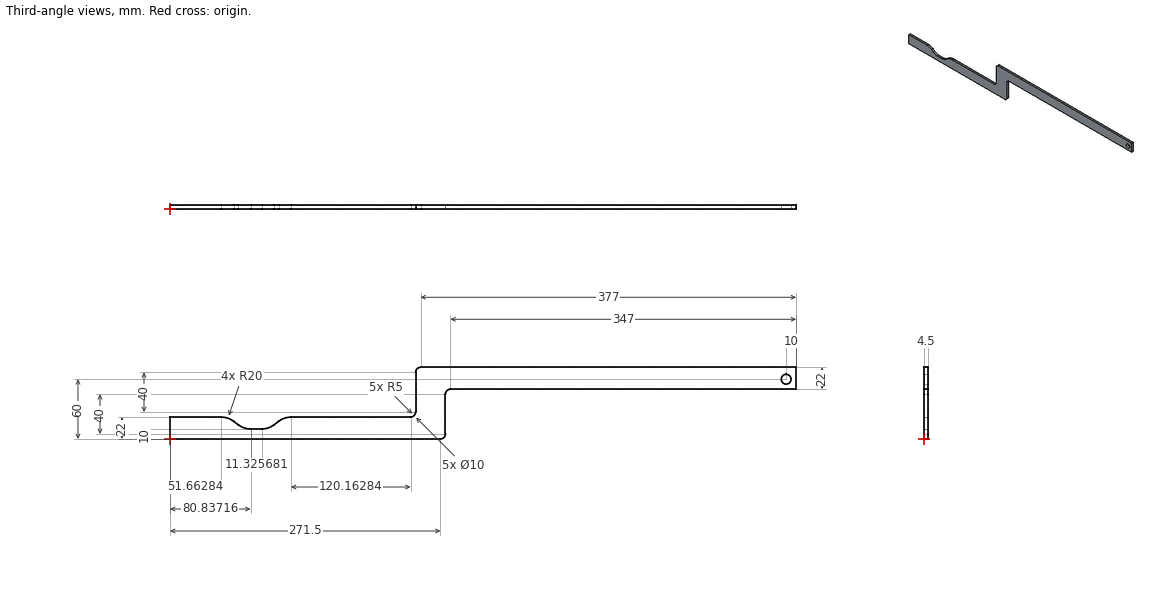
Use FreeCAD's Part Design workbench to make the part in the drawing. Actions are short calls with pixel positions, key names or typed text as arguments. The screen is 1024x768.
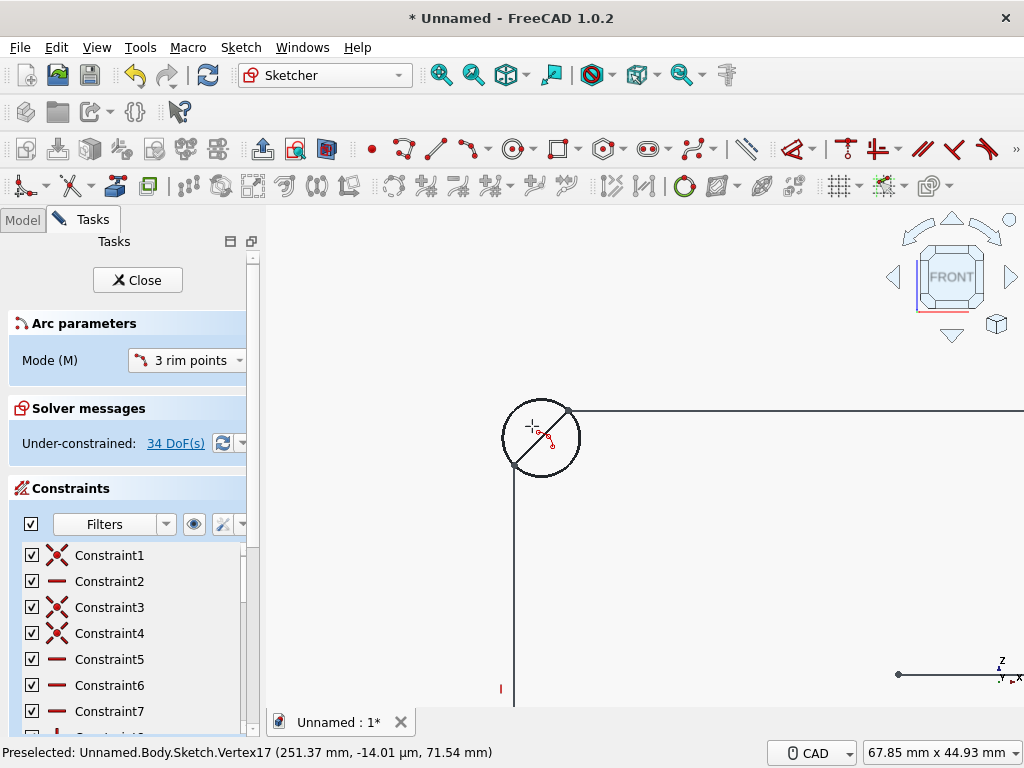
click(530, 422)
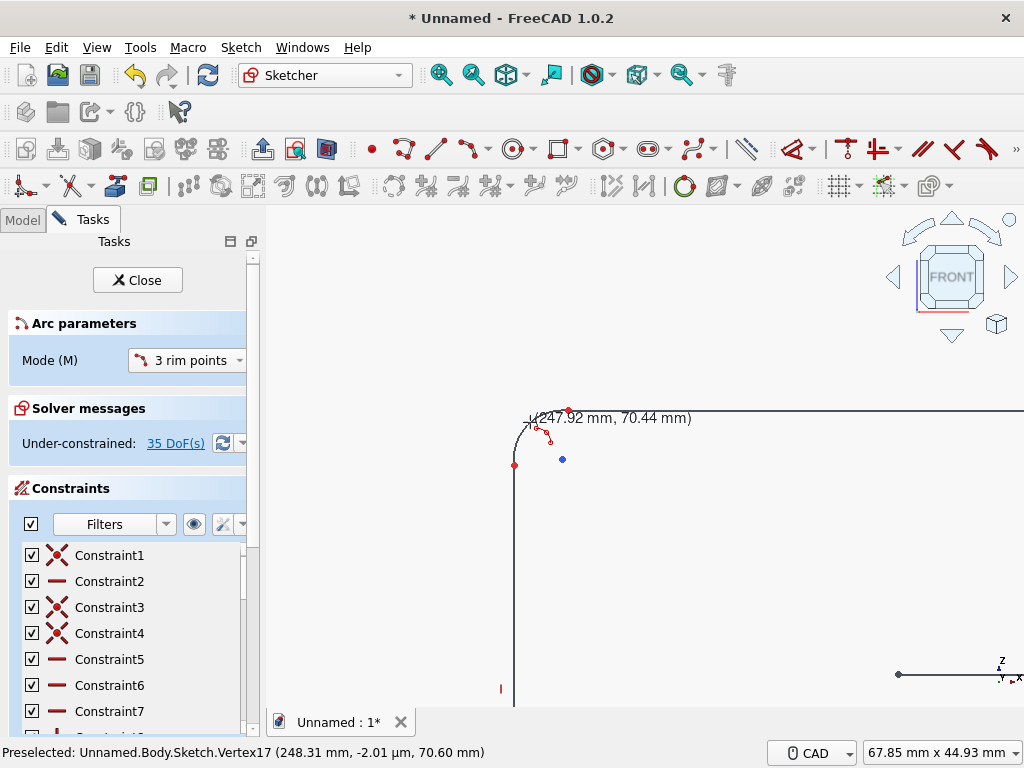
scroll(532, 433, down, 14)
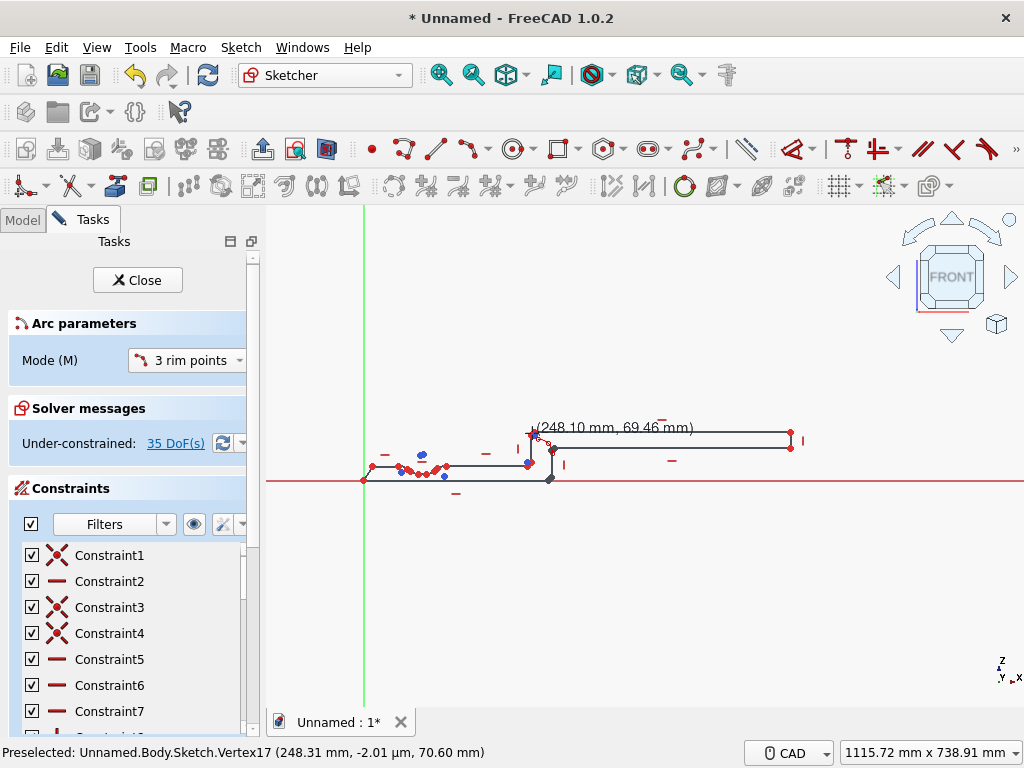
scroll(555, 447, up, 6)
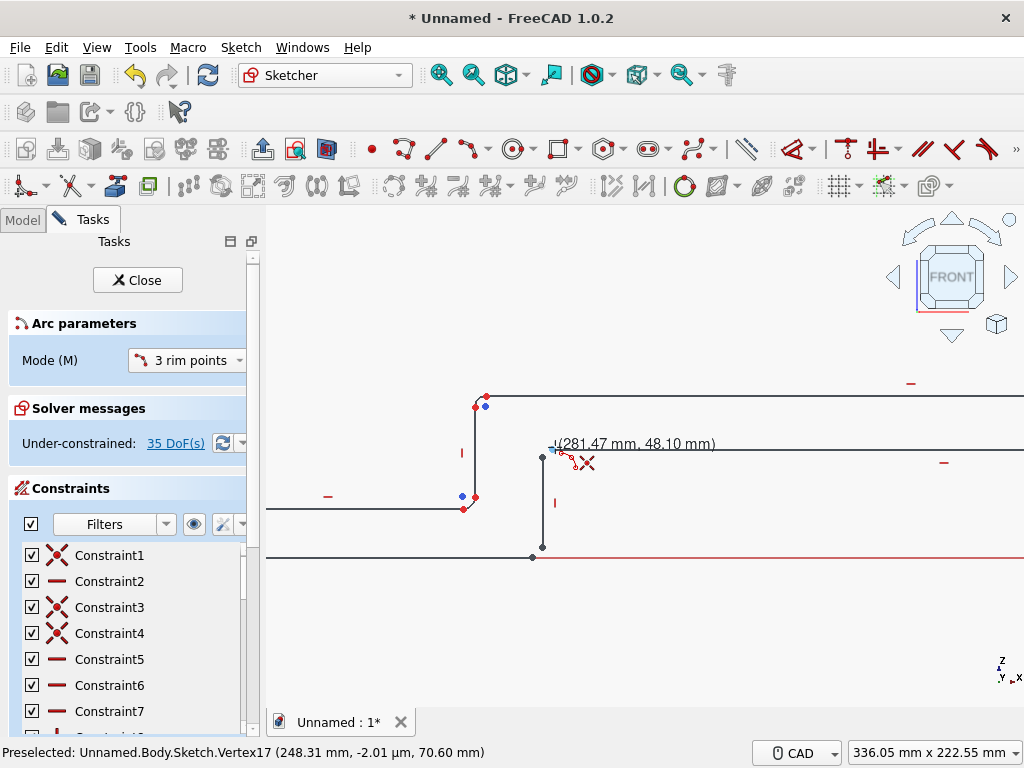
click(553, 450)
click(543, 457)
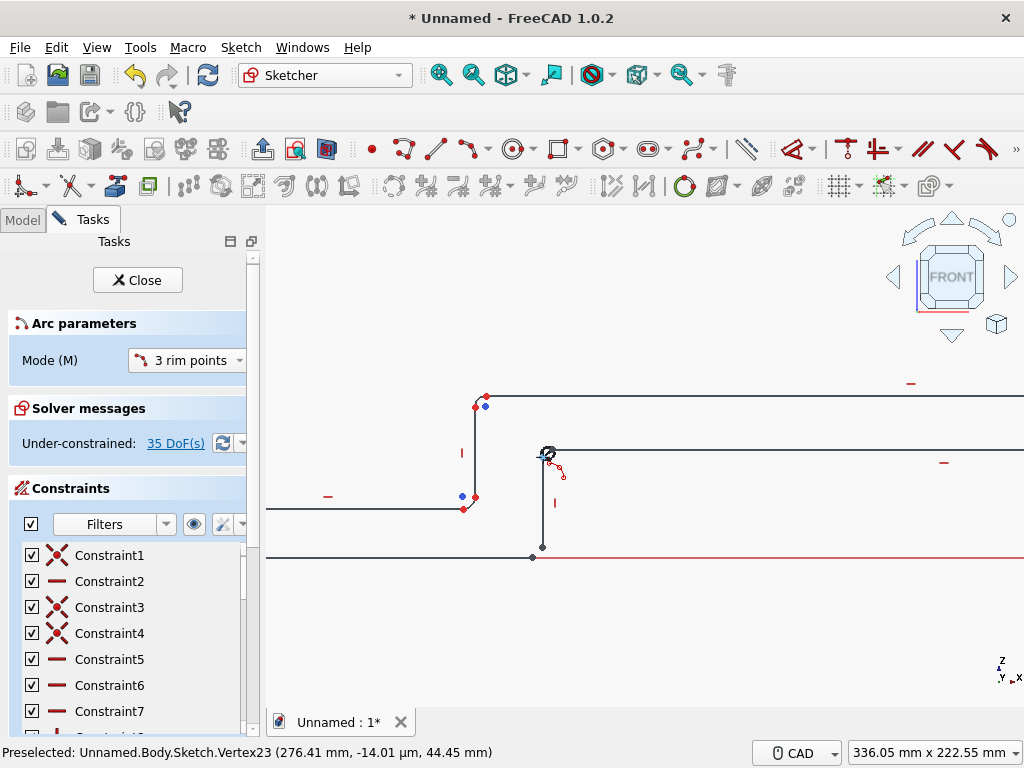
scroll(546, 448, up, 8)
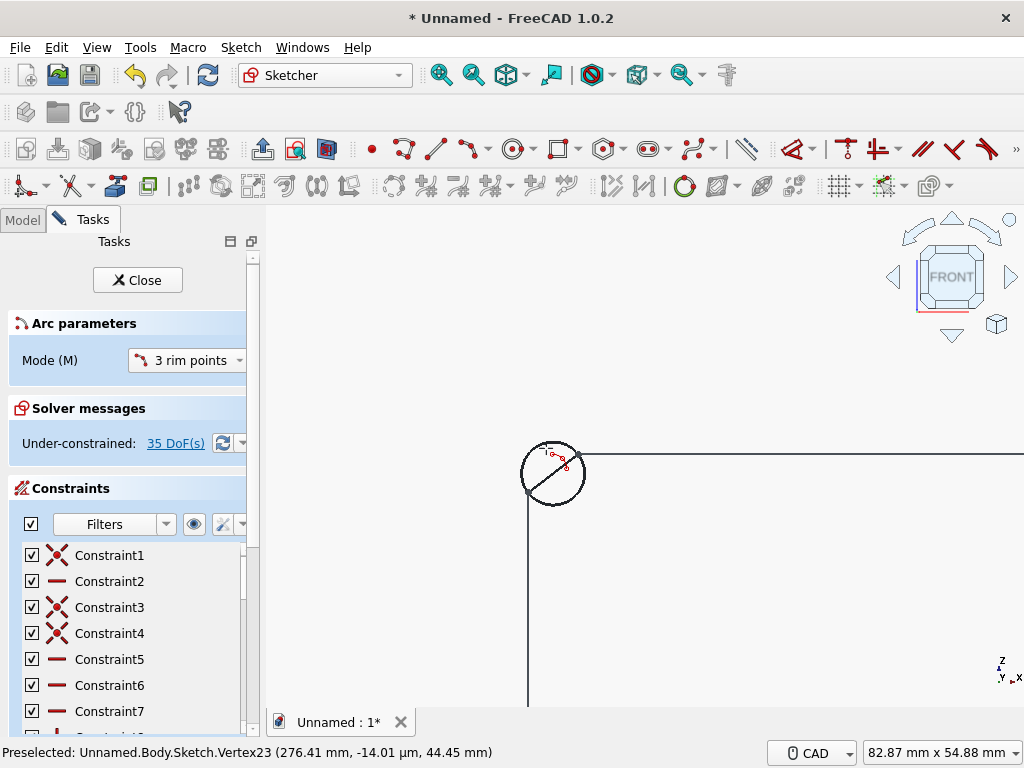
click(546, 447)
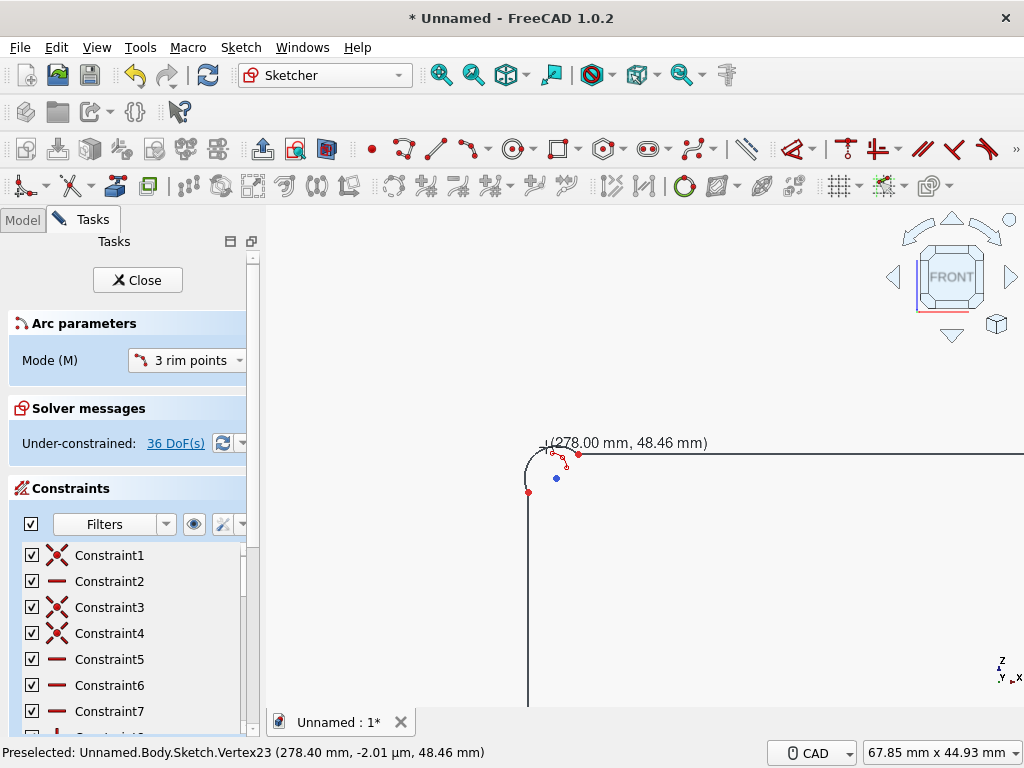
scroll(552, 448, down, 14)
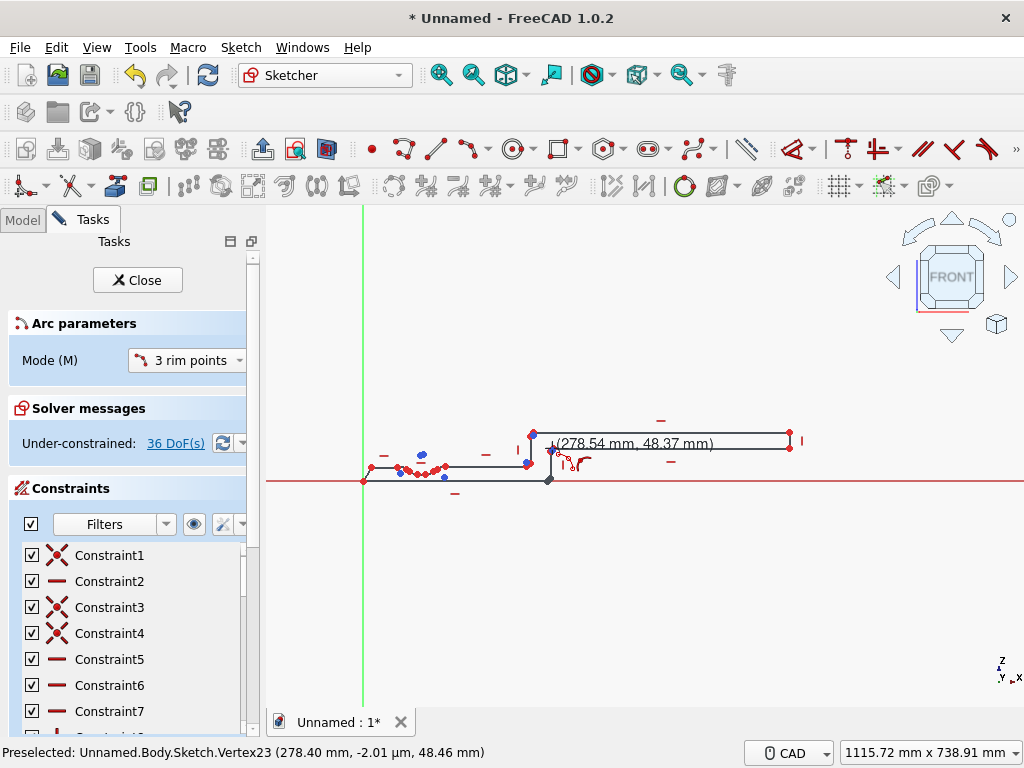
scroll(551, 478, up, 8)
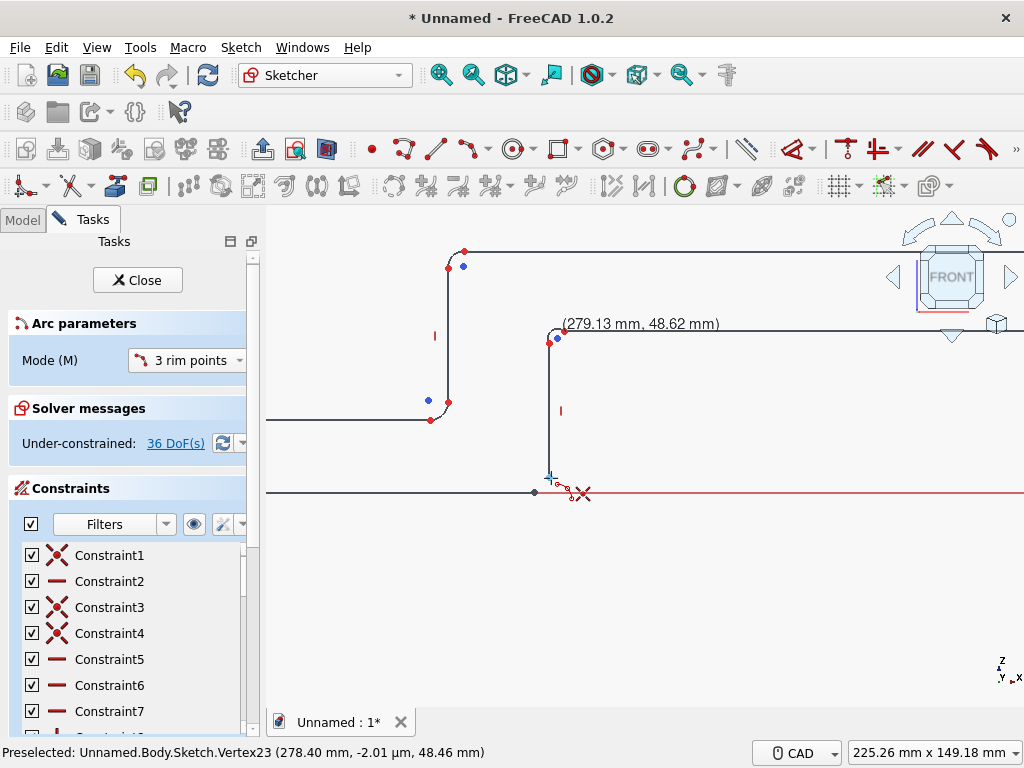
click(549, 477)
click(534, 493)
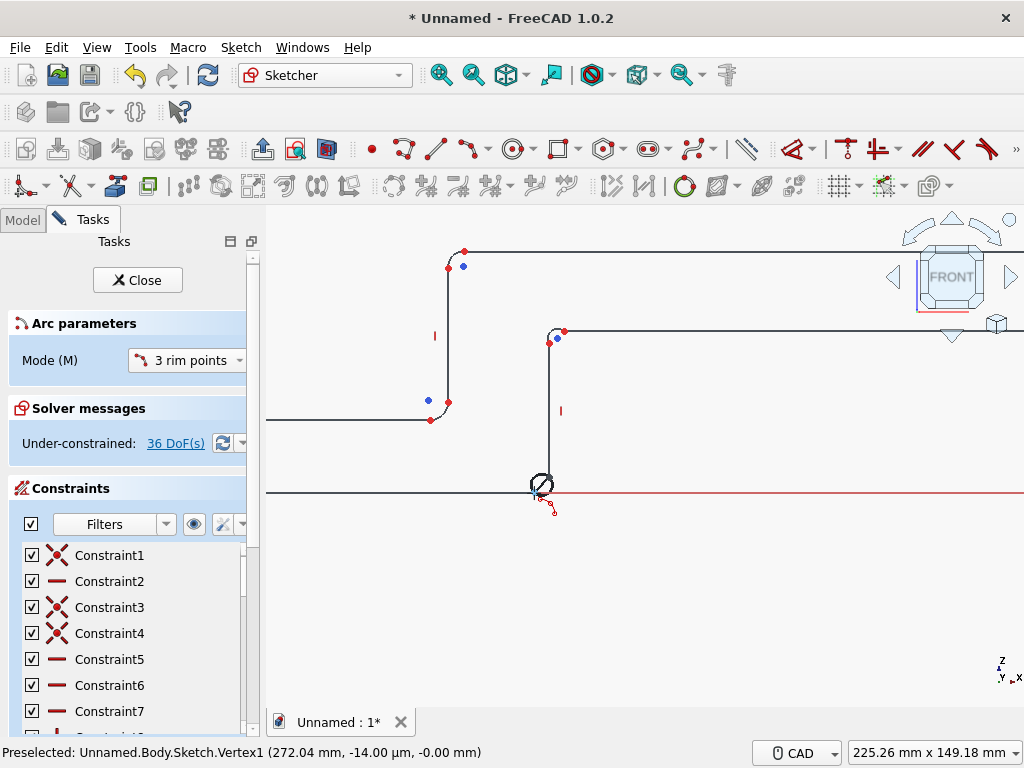
scroll(544, 488, up, 6)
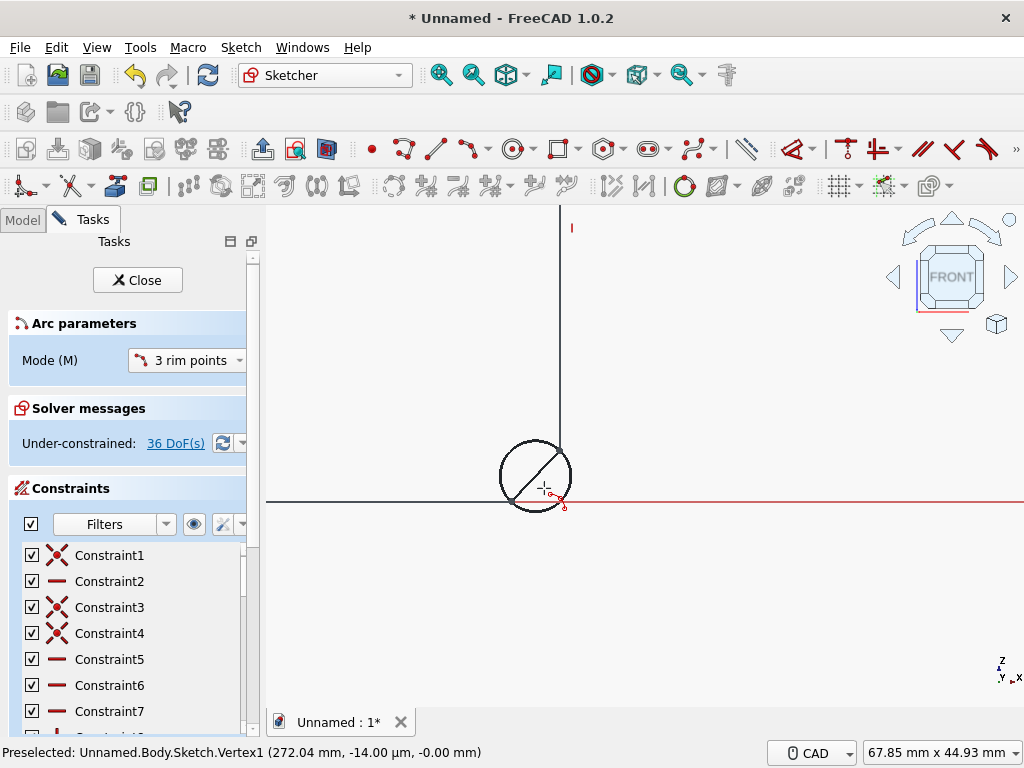
click(545, 486)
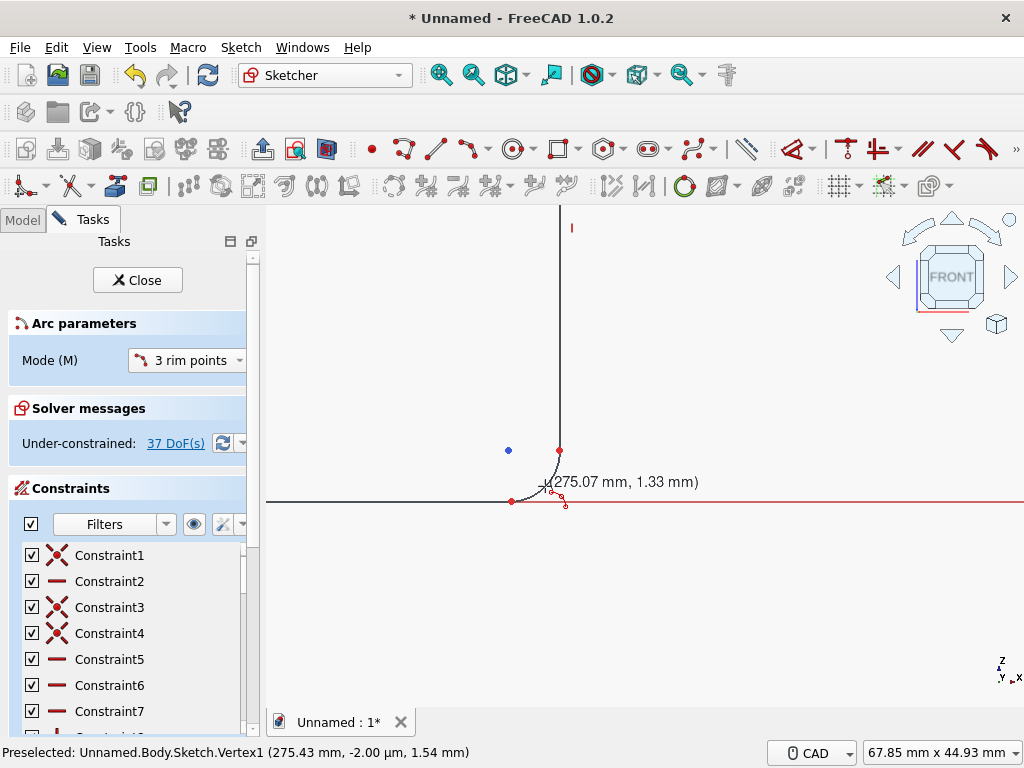
click(514, 150)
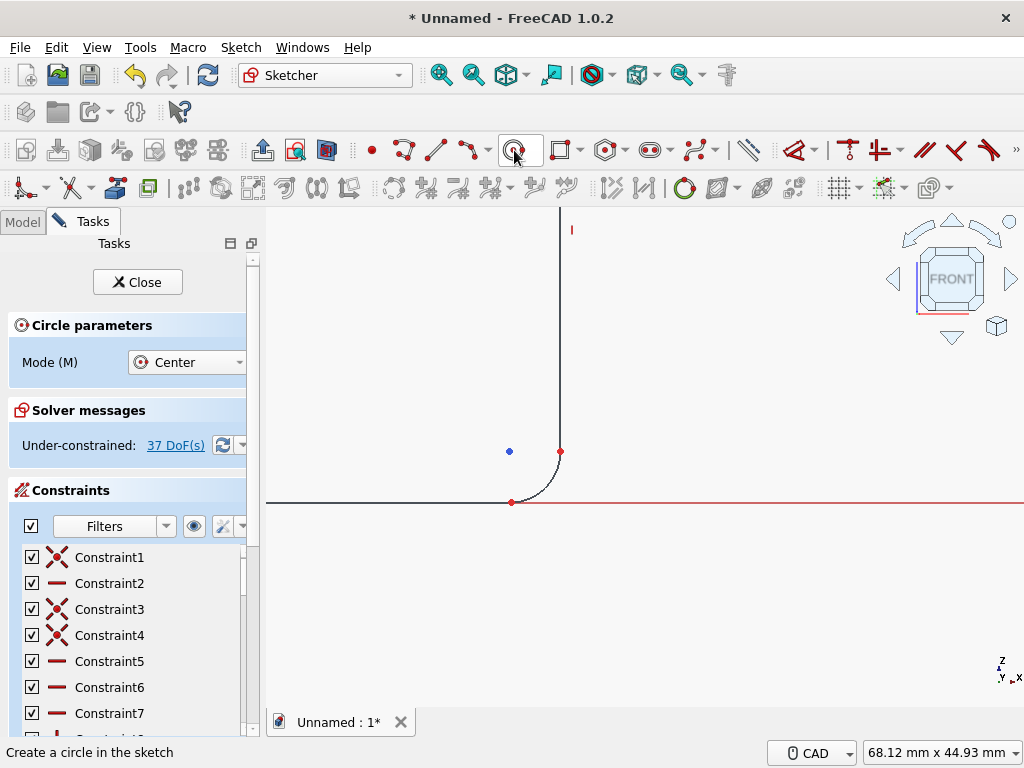
scroll(550, 480, down, 14)